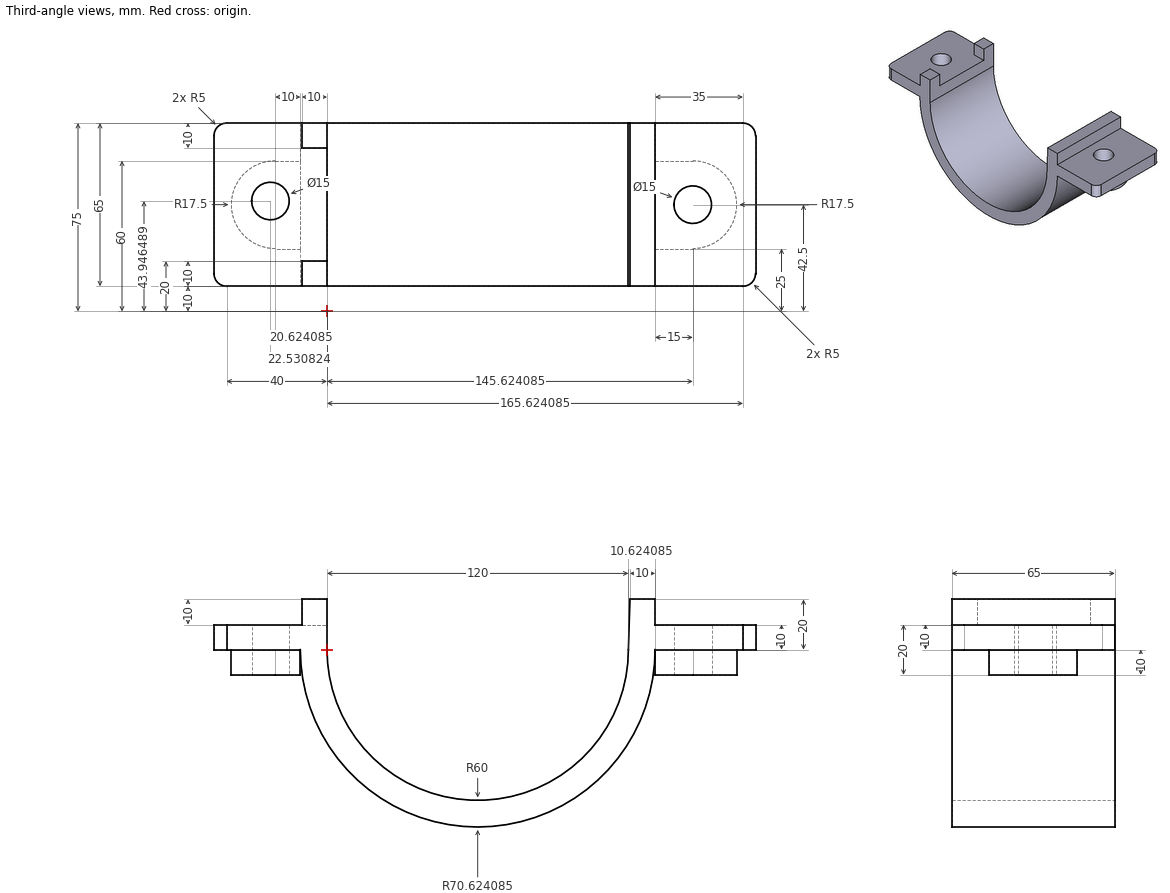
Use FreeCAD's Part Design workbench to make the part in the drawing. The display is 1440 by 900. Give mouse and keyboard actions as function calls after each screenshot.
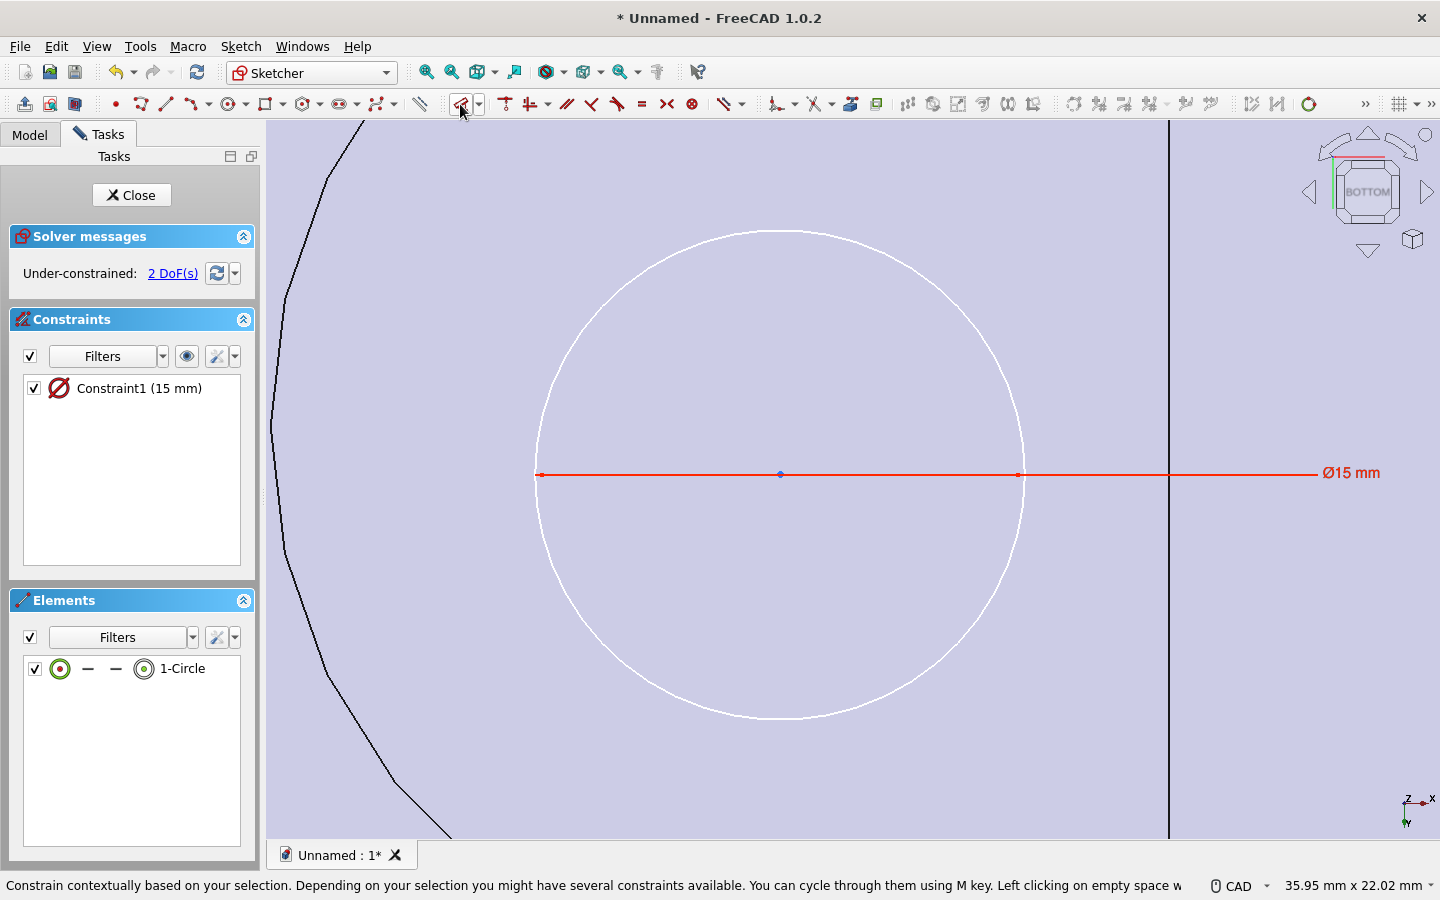
click(780, 475)
click(914, 509)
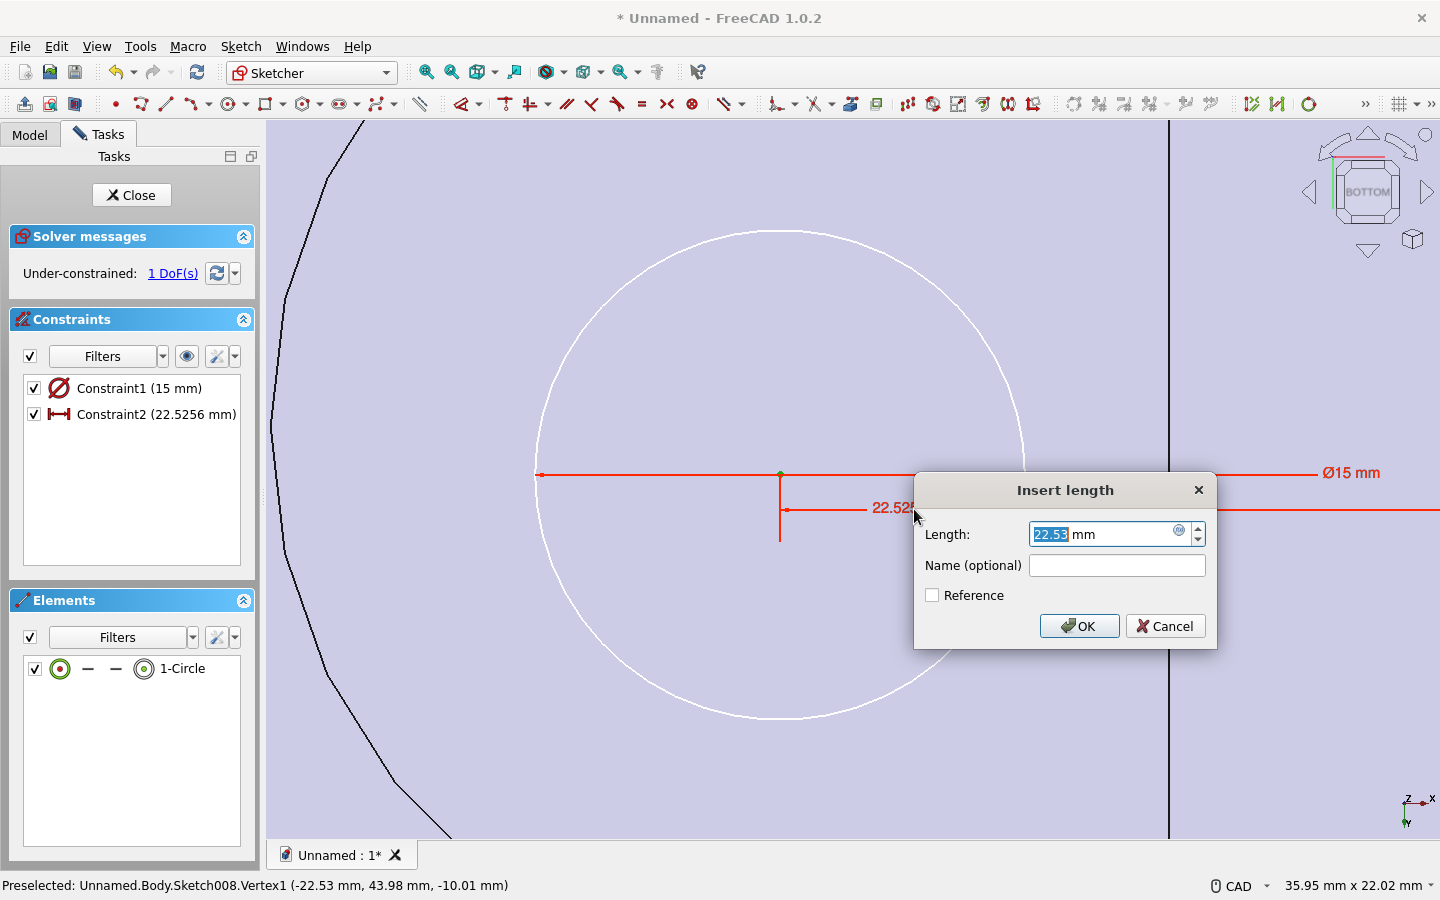
text(22.530824)
key(Return)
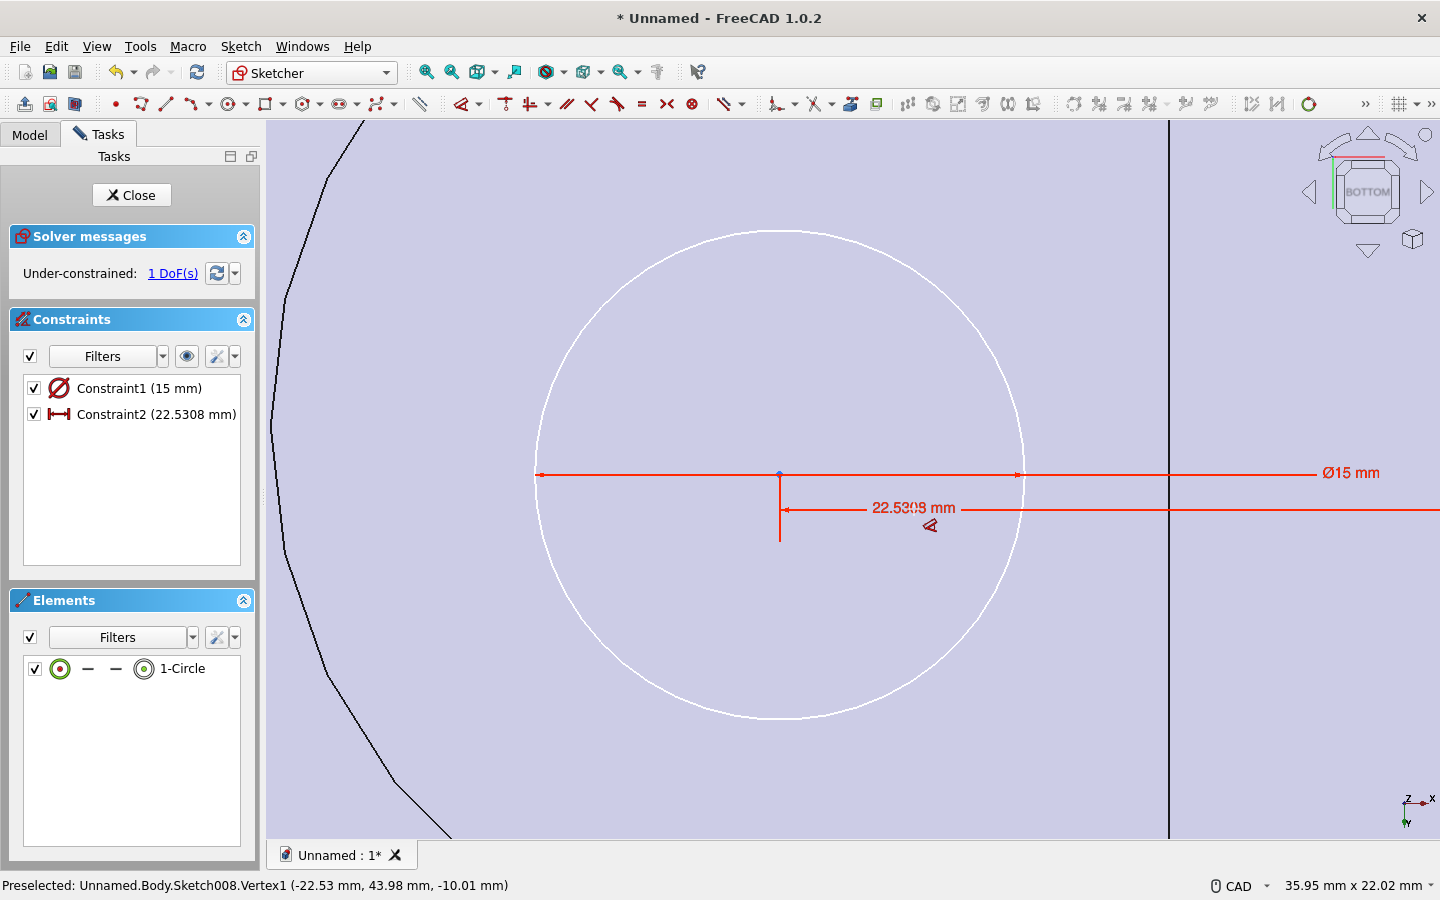
click(780, 475)
click(746, 312)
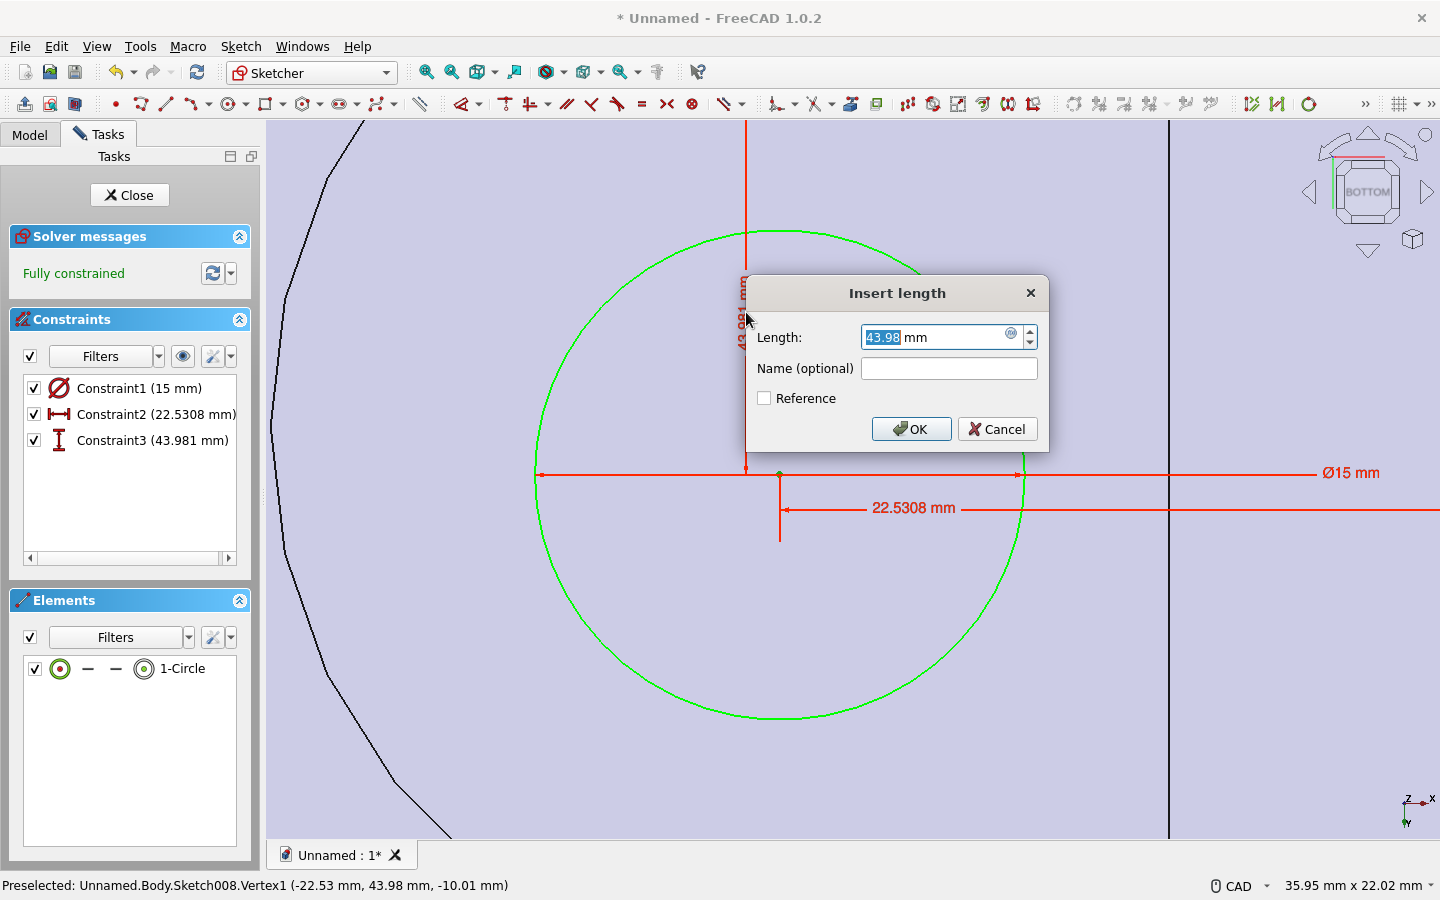
text(43.946489)
key(Return)
key(Escape)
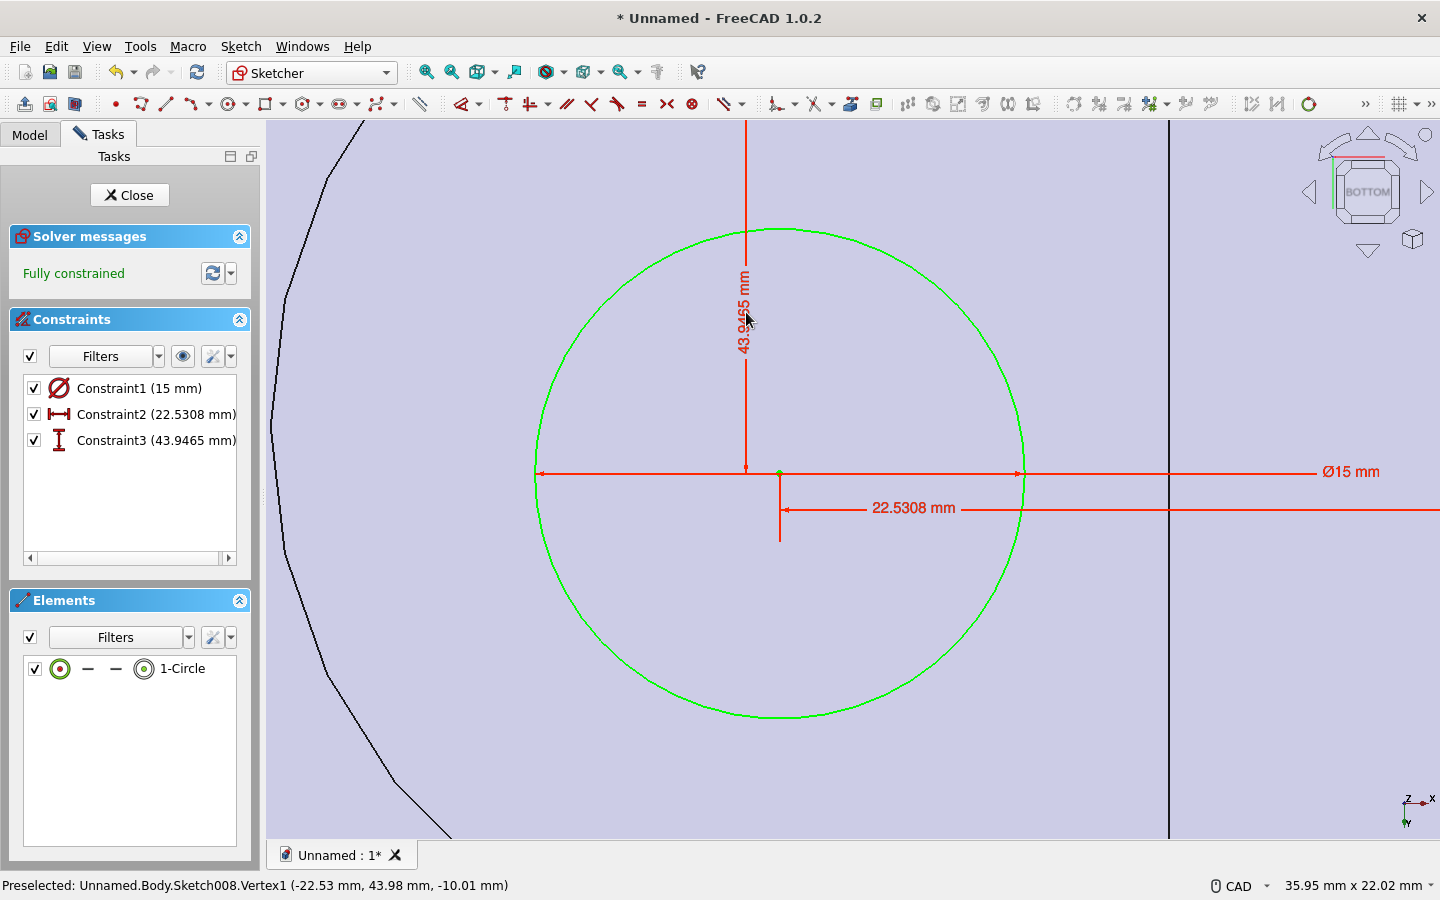
click(130, 195)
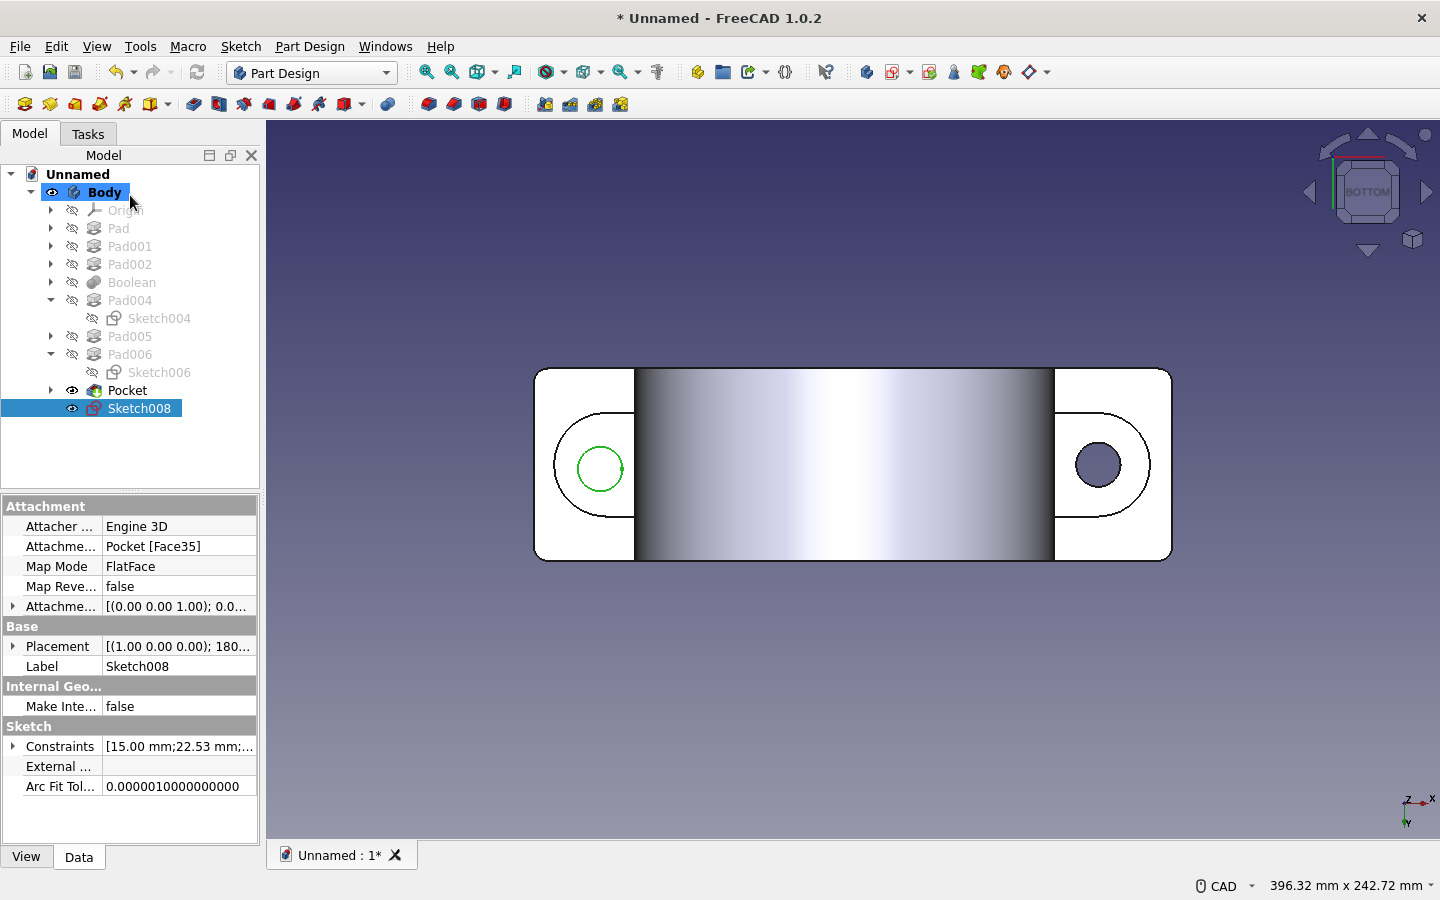
click(194, 104)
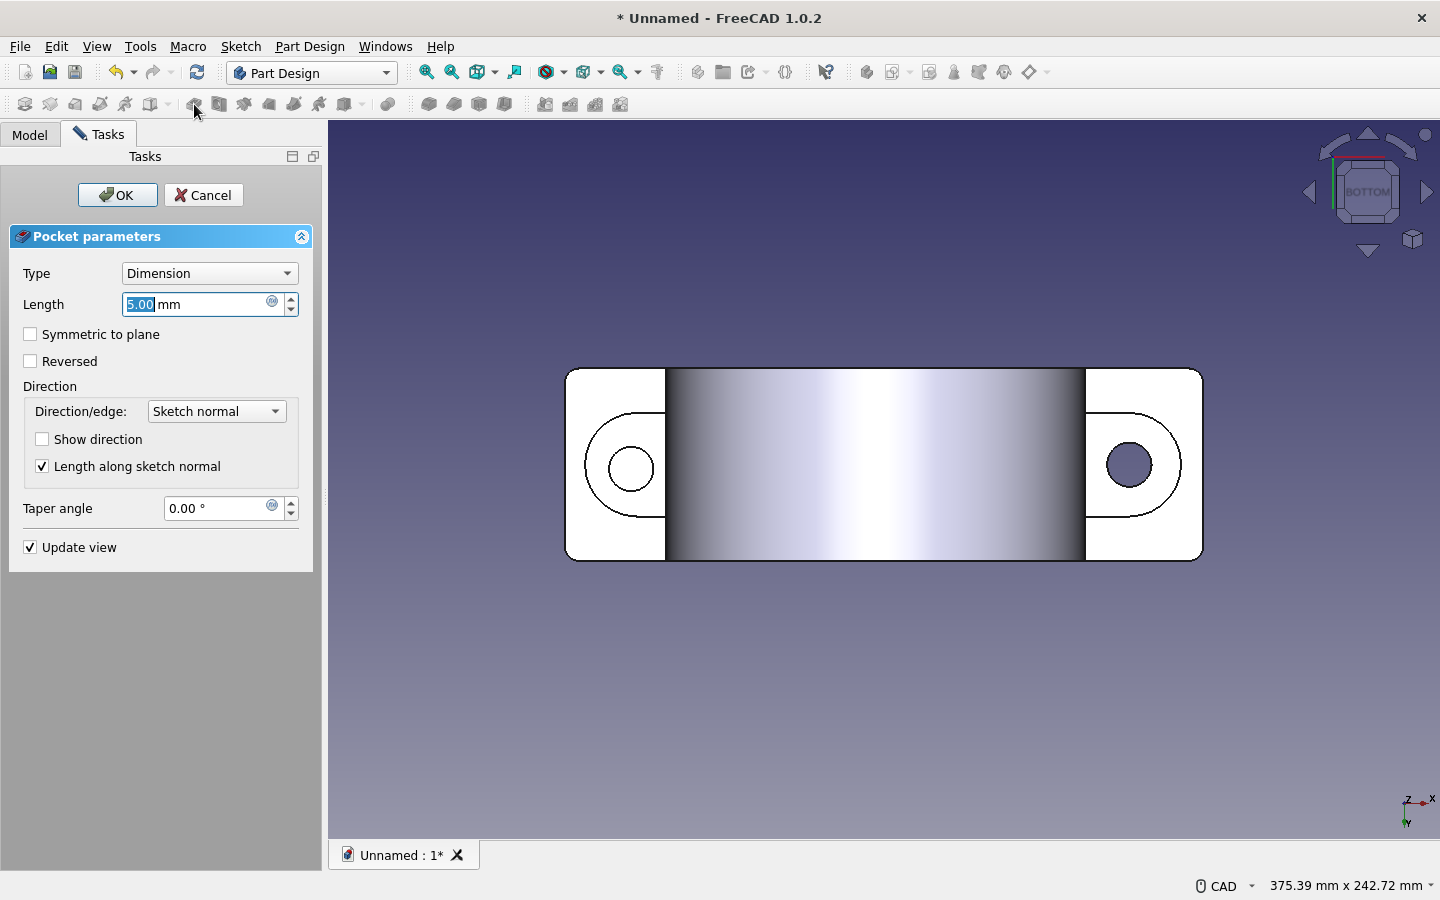
text(20)
key(Tab)